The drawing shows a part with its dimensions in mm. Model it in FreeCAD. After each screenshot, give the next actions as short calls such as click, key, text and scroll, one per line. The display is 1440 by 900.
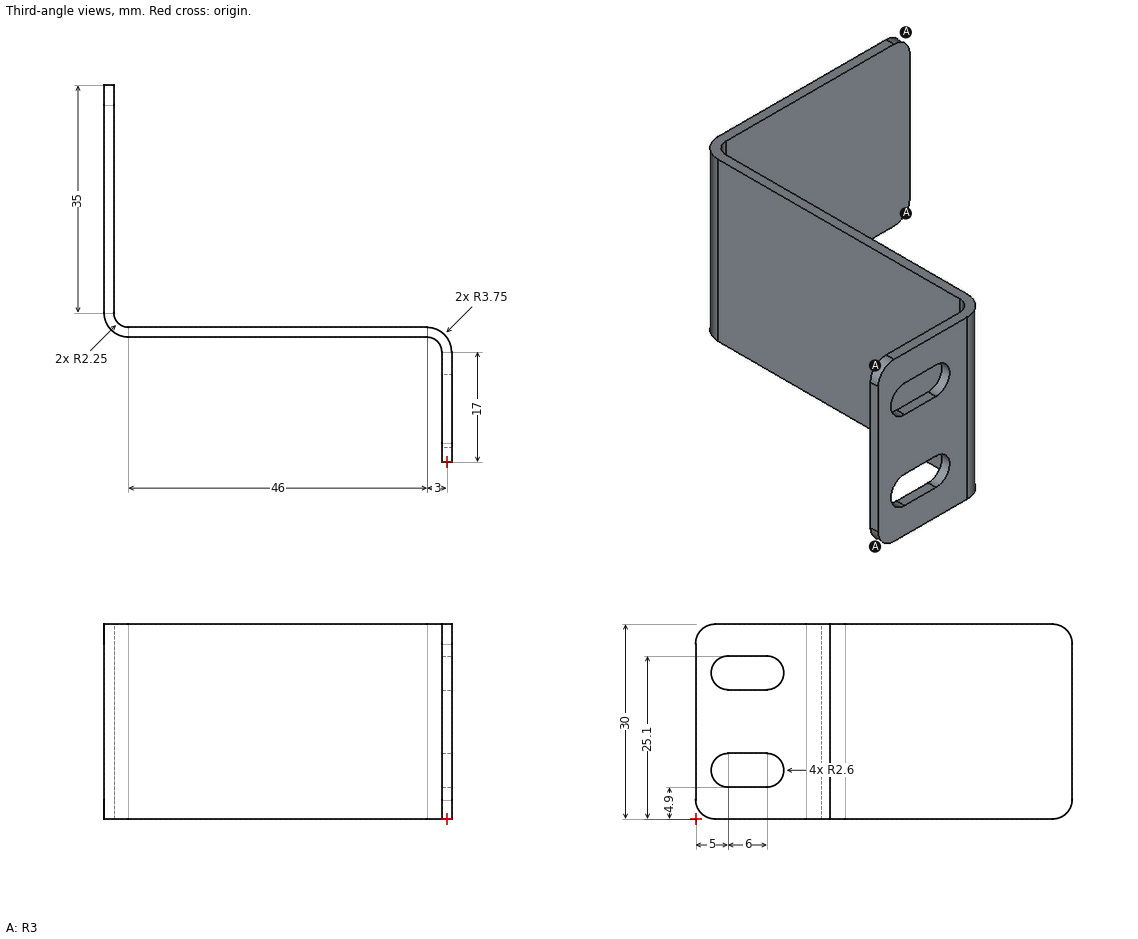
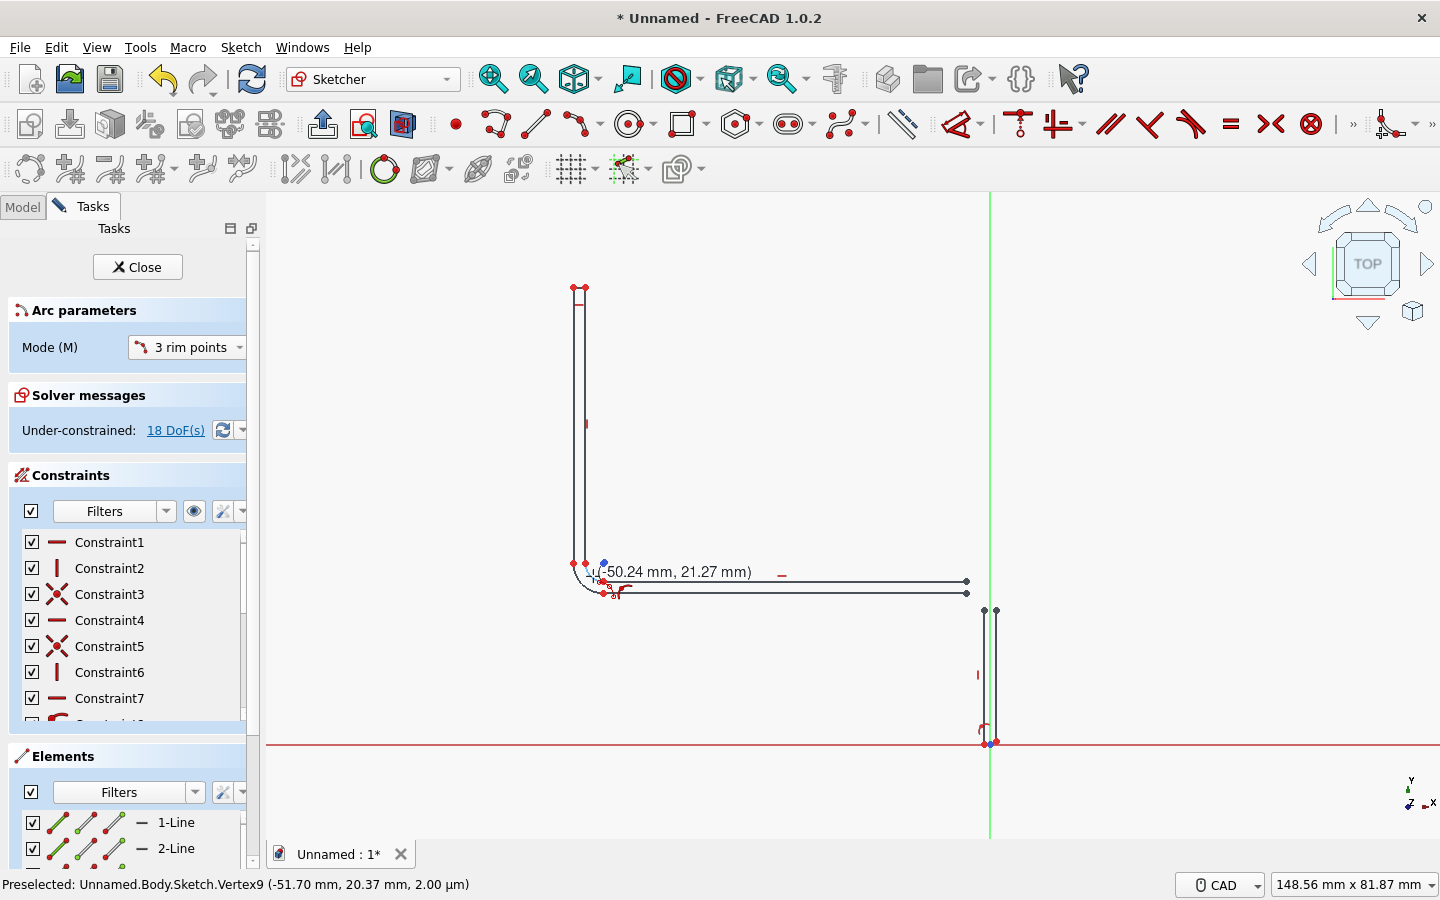
scroll(967, 593, up, 2)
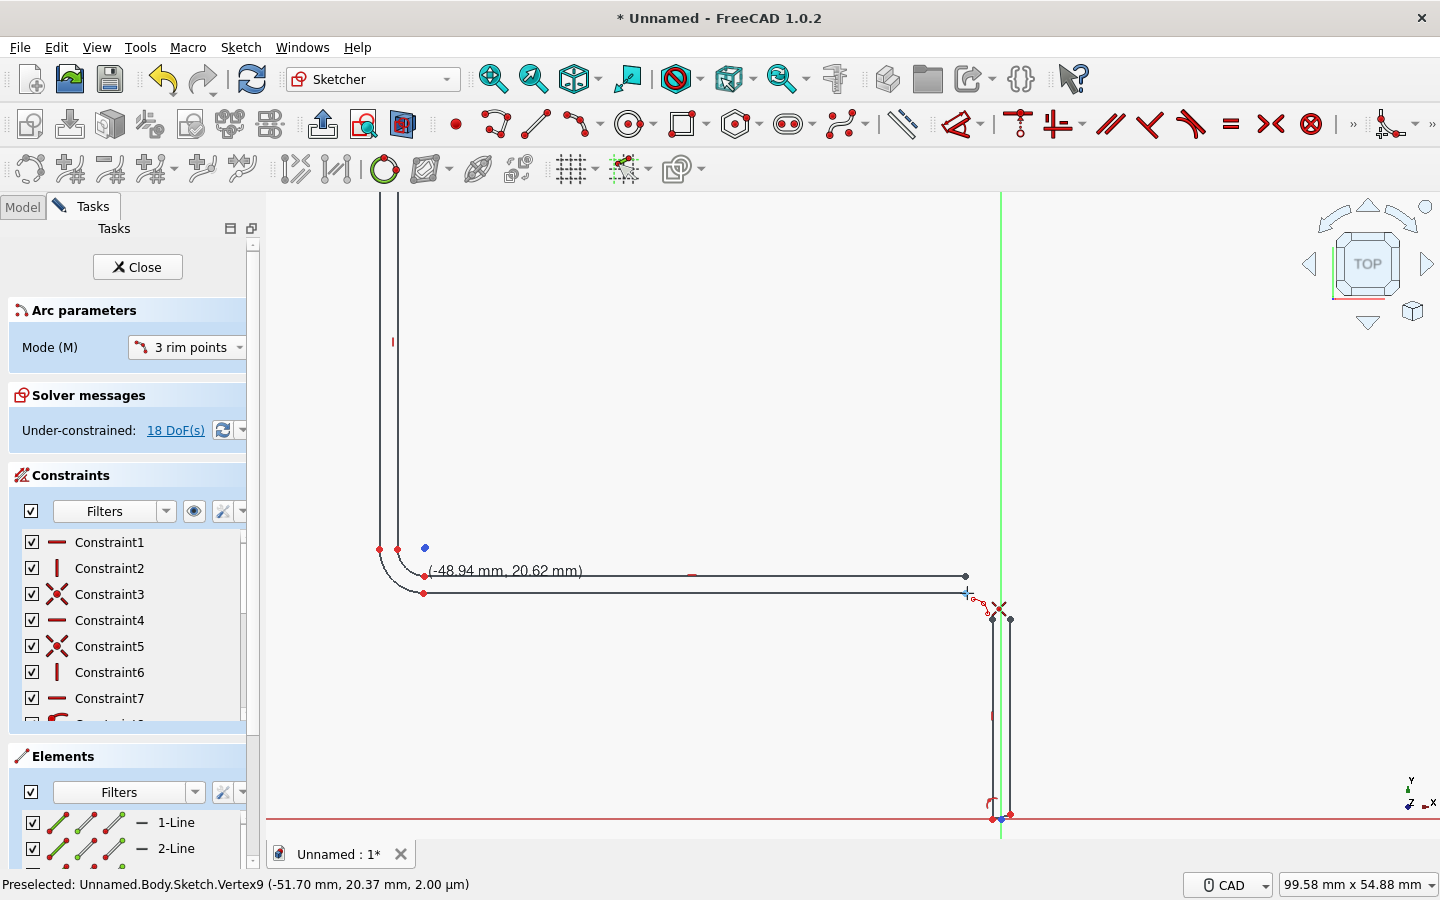
click(966, 593)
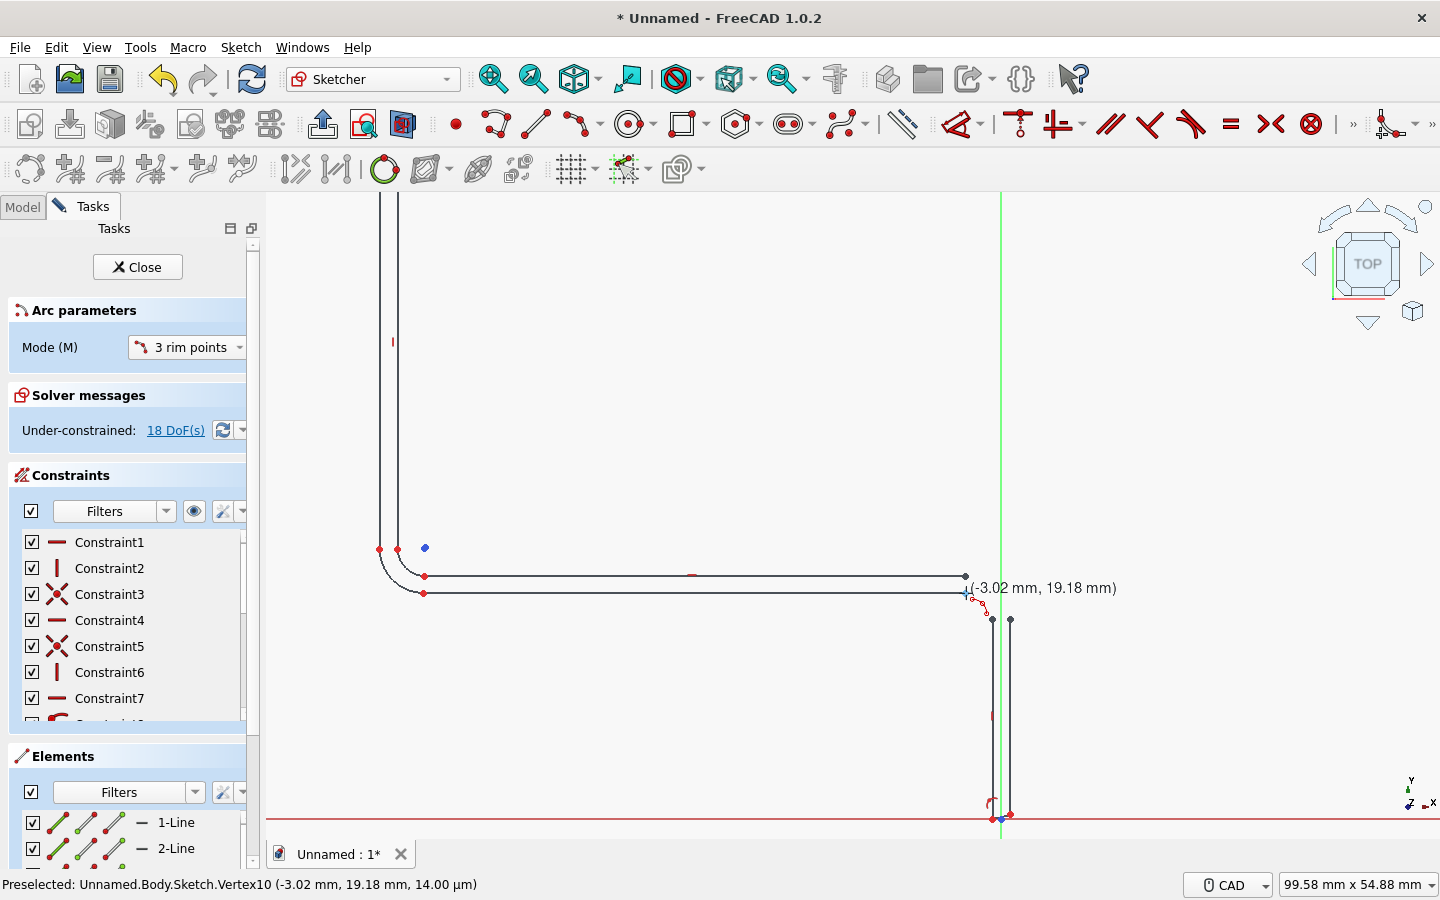
scroll(993, 619, up, 3)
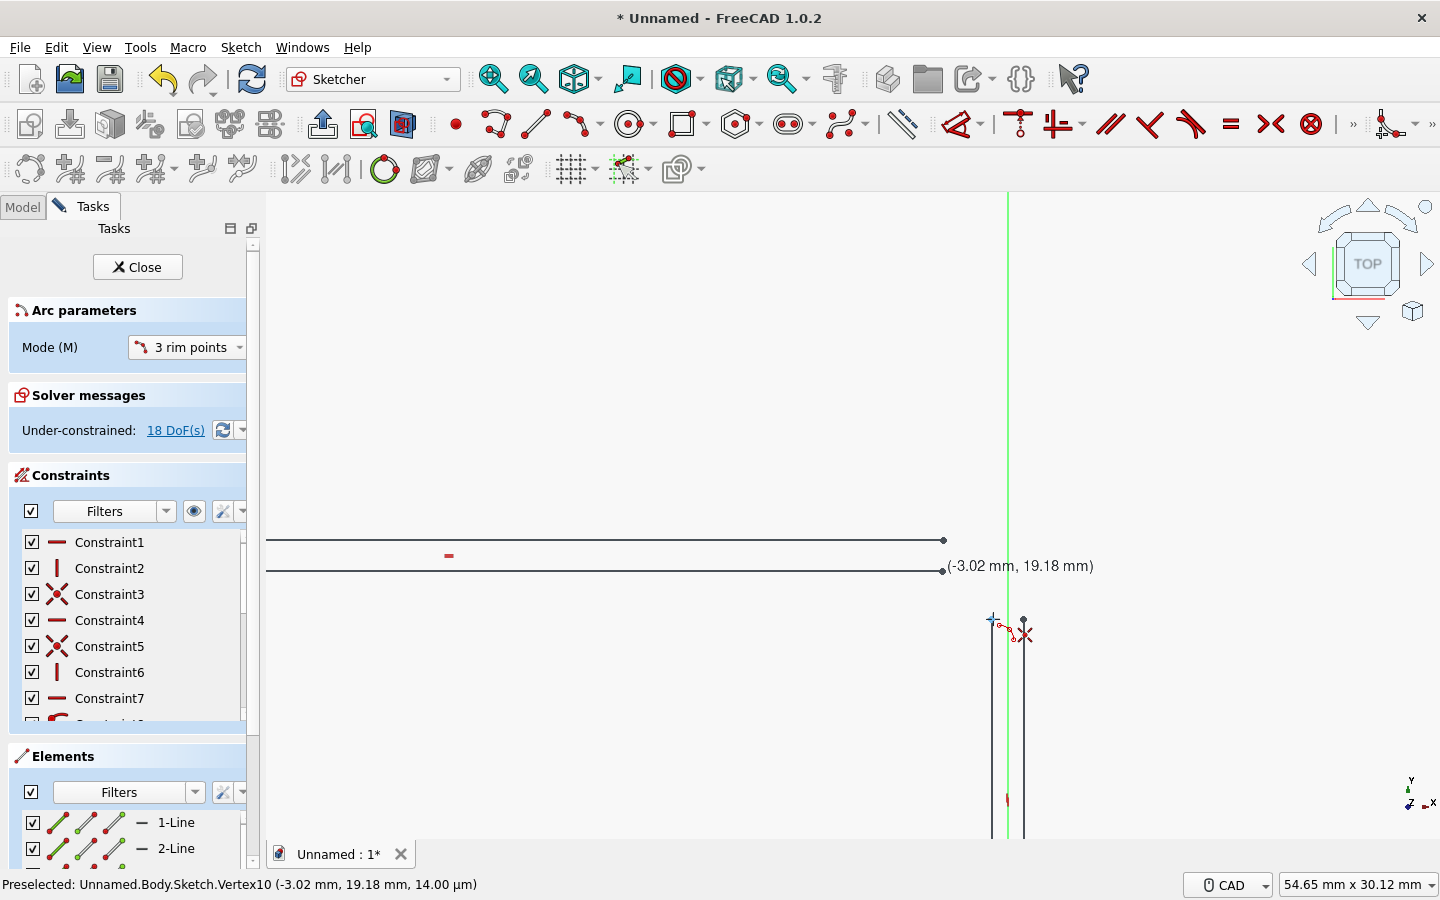
click(992, 619)
click(977, 584)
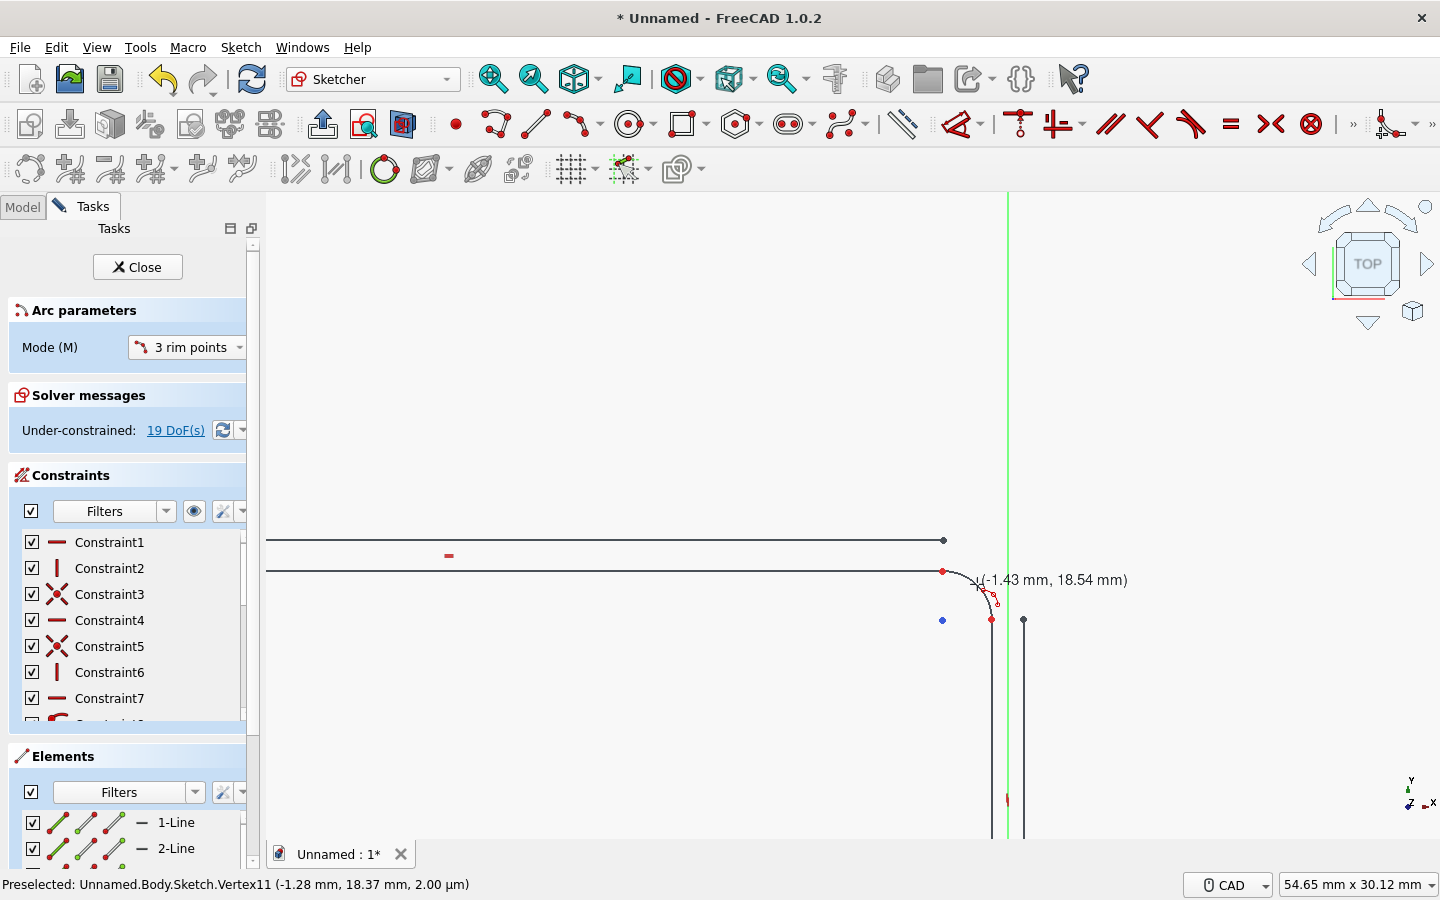
click(1024, 619)
click(943, 540)
click(980, 546)
key(Escape)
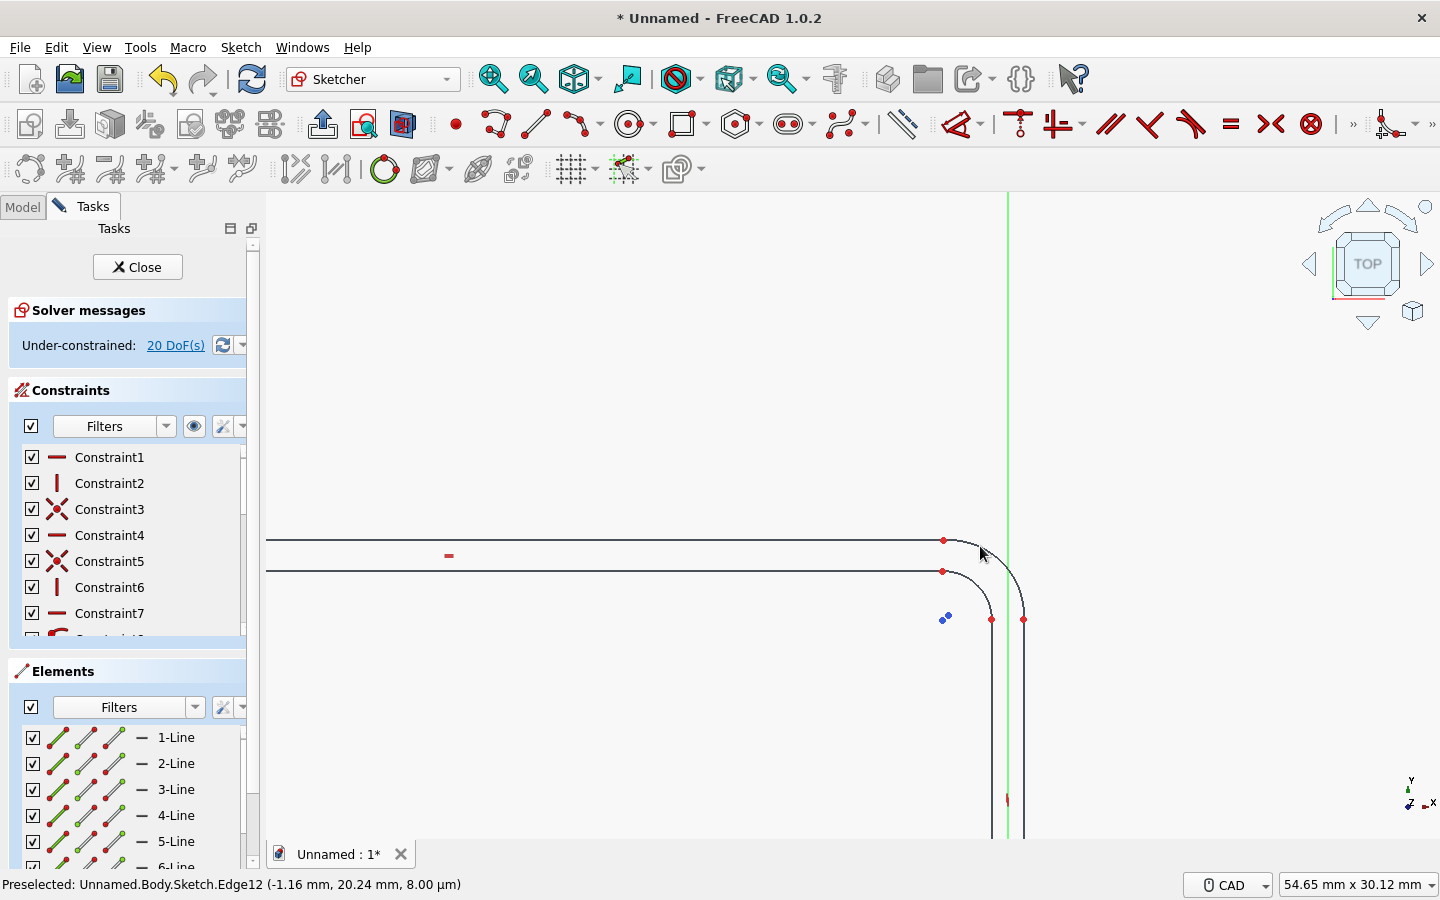
click(647, 540)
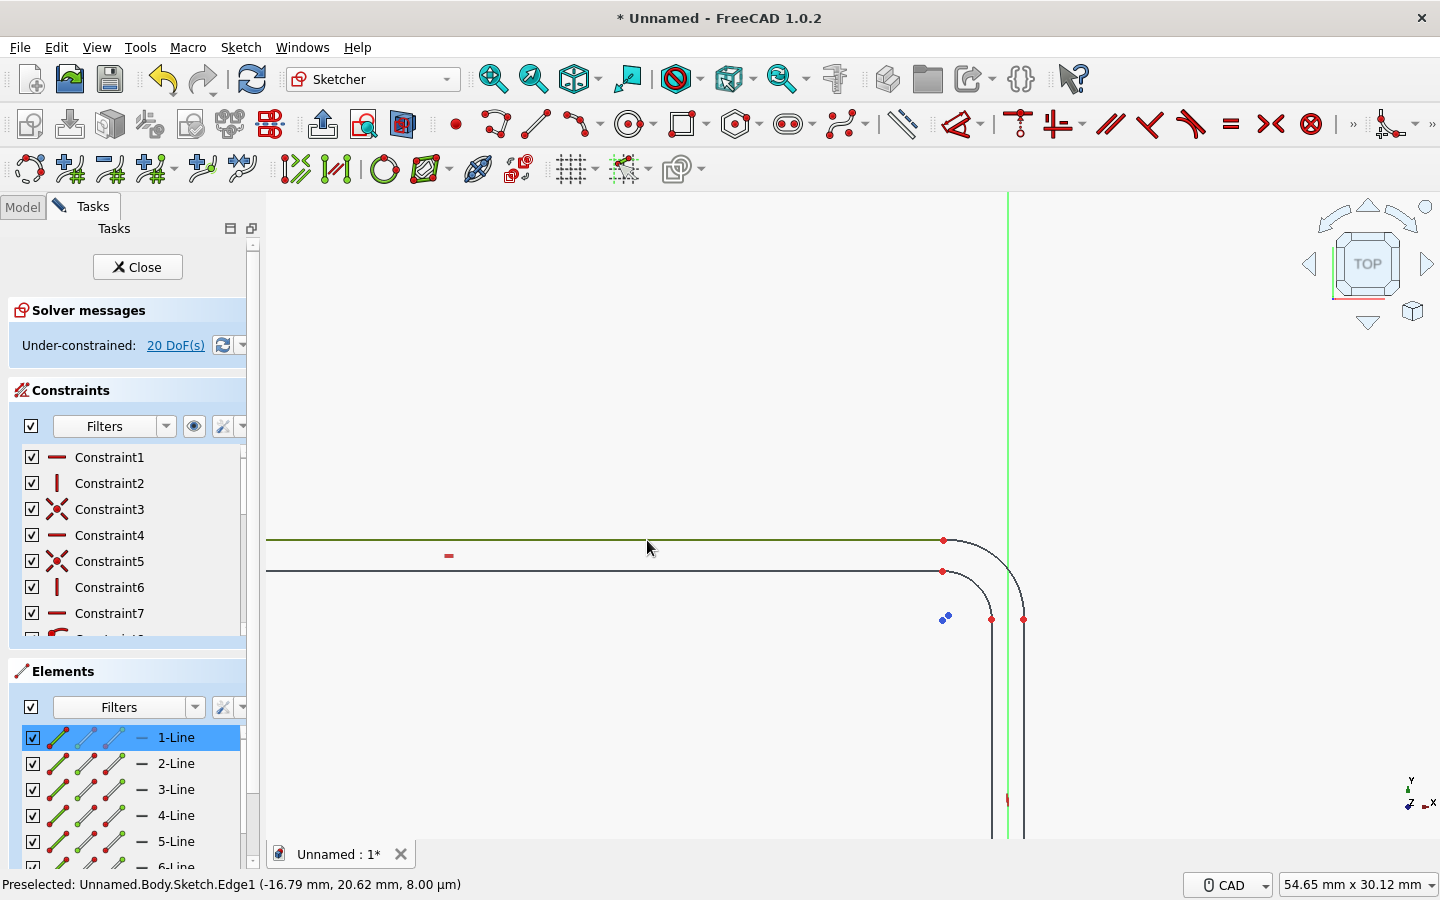
scroll(980, 606, down, 5)